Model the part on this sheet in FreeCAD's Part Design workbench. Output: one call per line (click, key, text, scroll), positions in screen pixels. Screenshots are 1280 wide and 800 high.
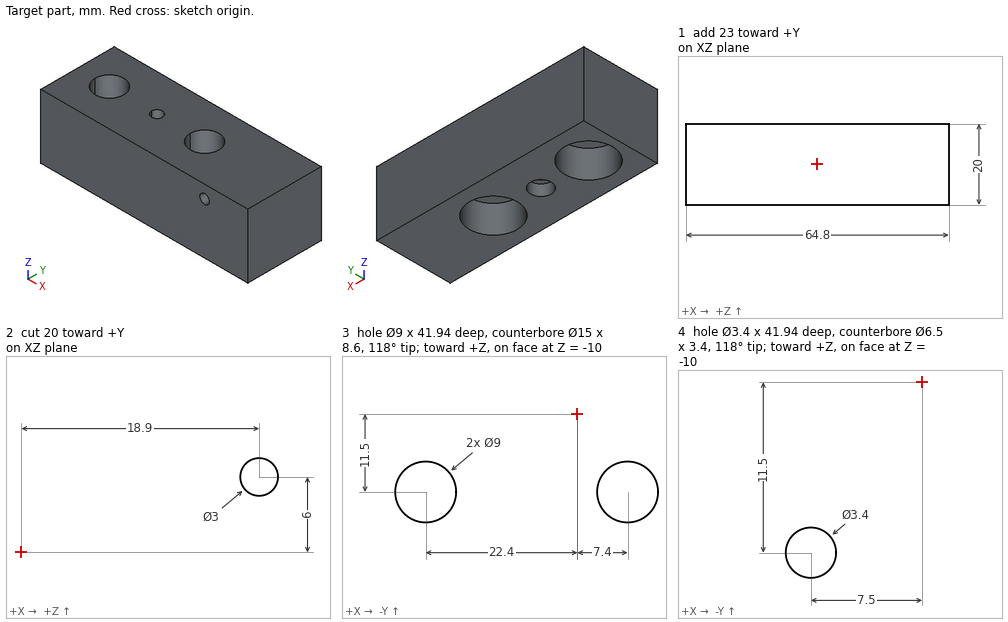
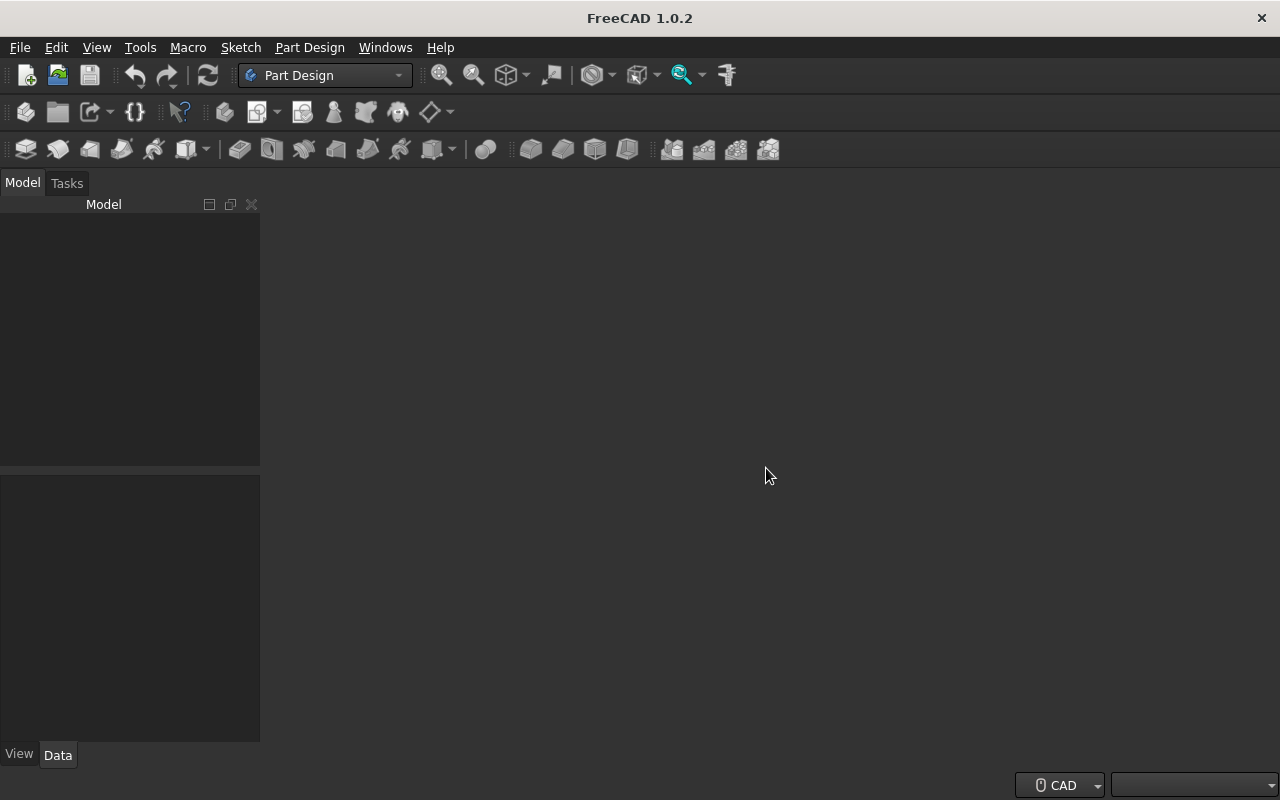
click(26, 76)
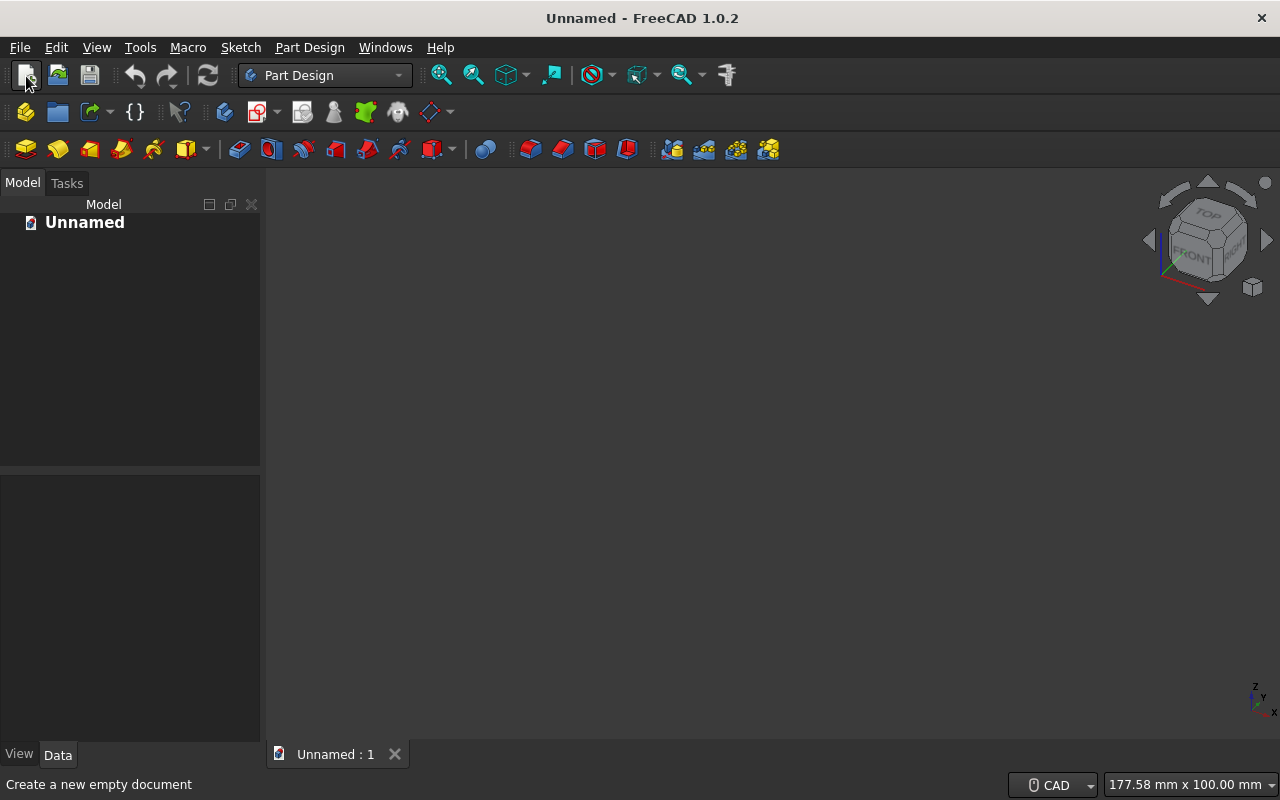
click(258, 112)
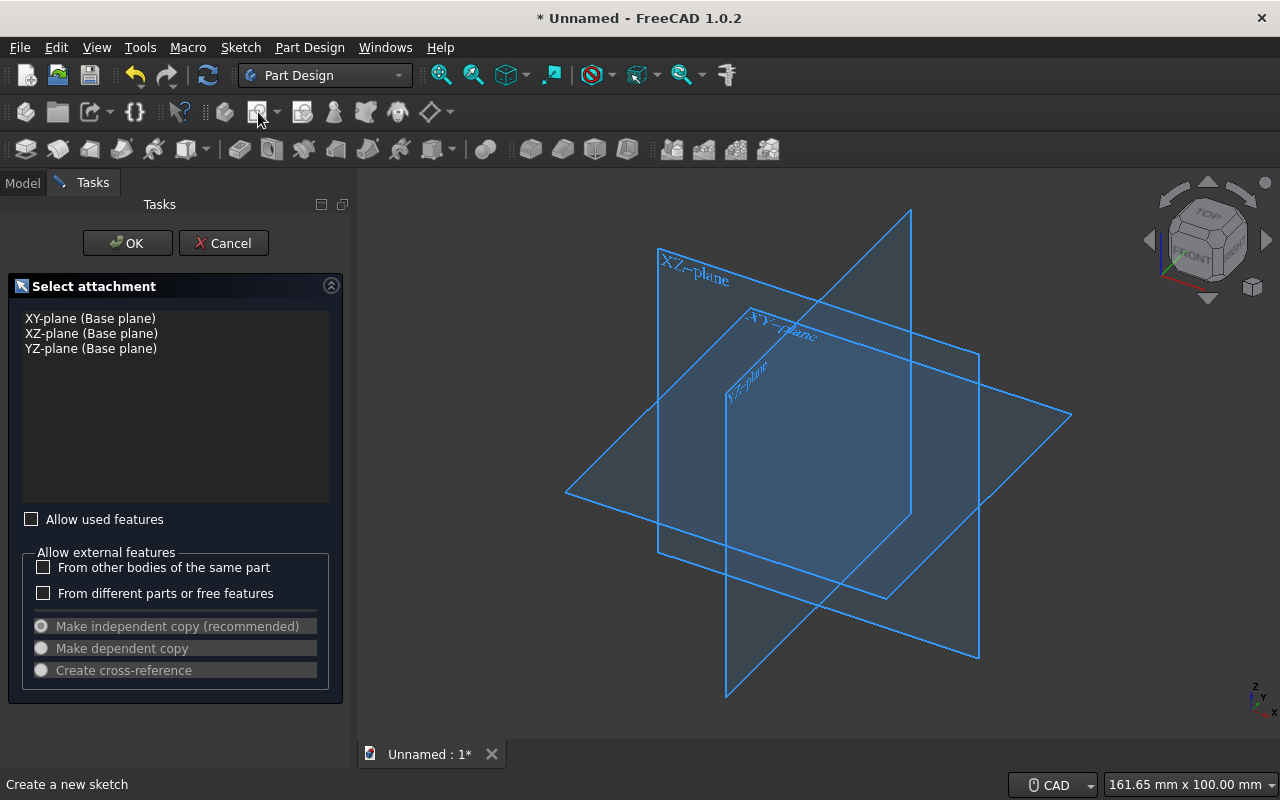
click(82, 334)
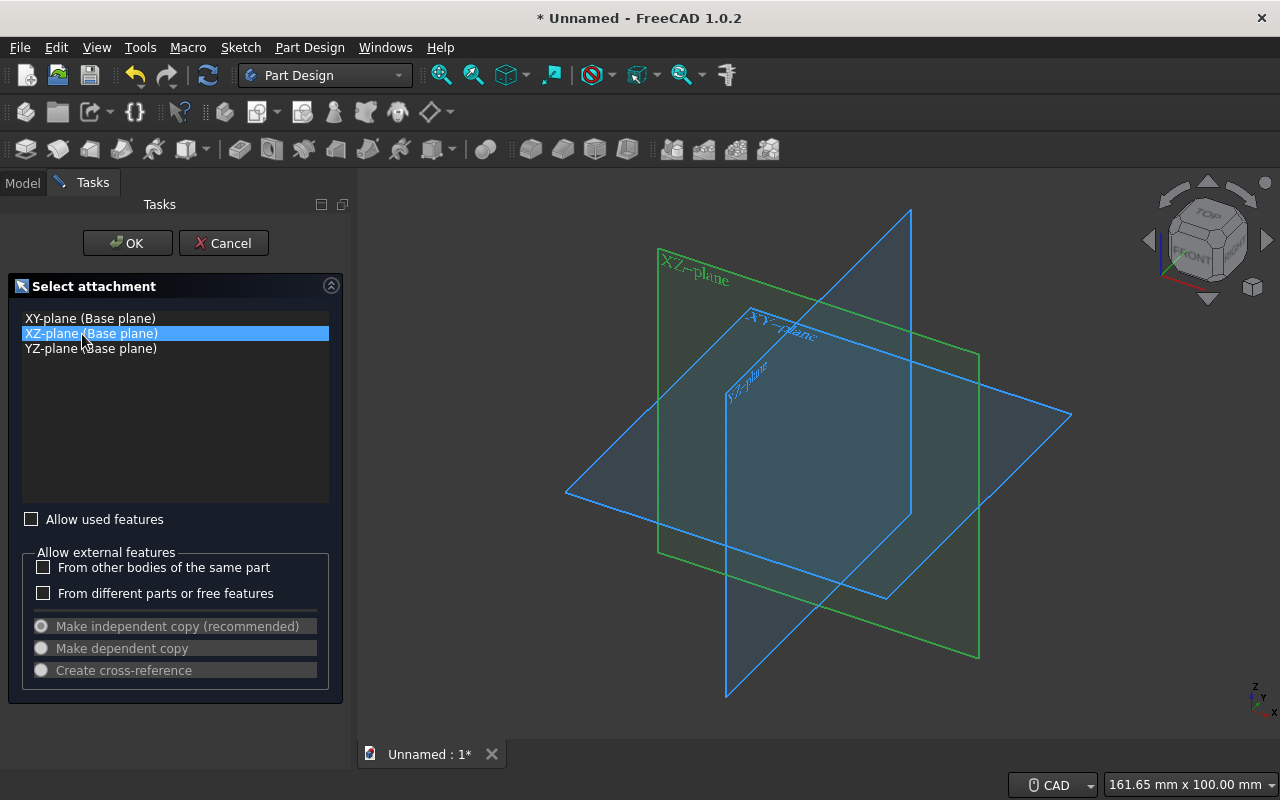
click(128, 243)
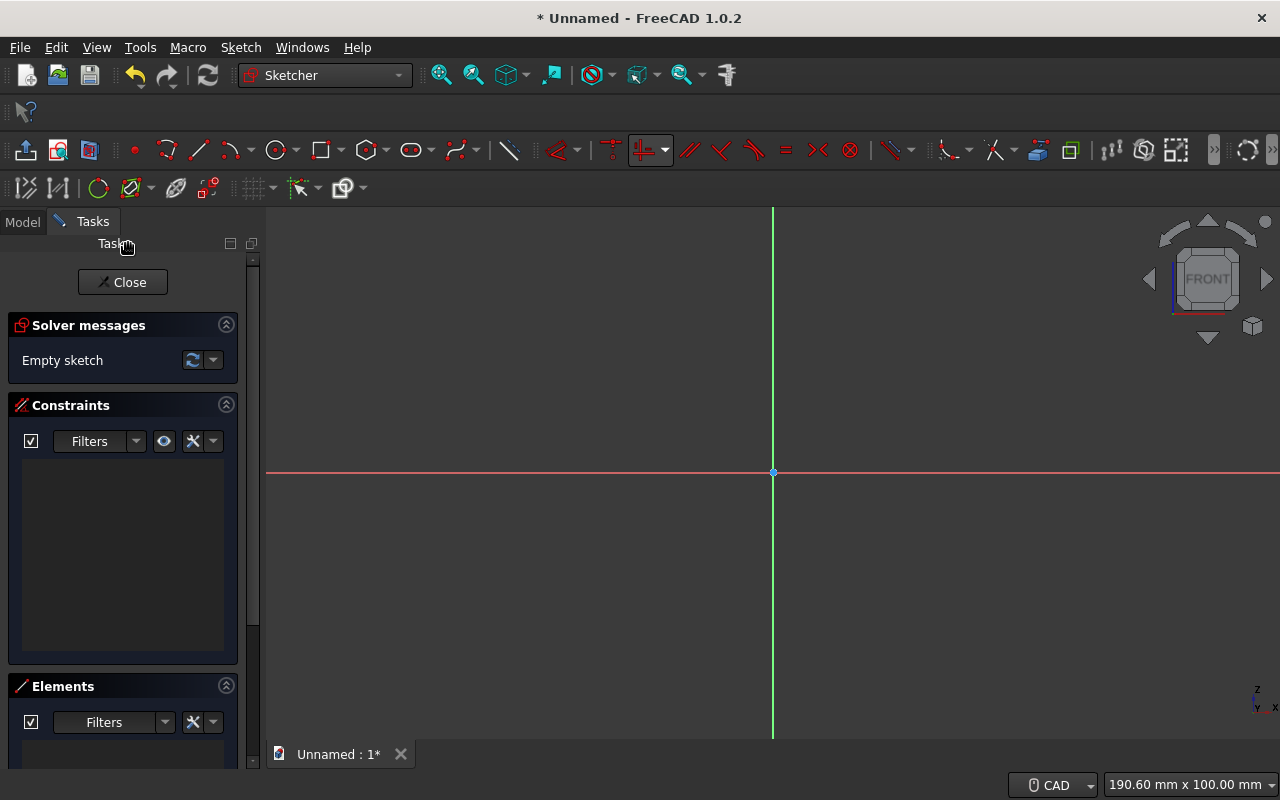
scroll(856, 473, up, 3)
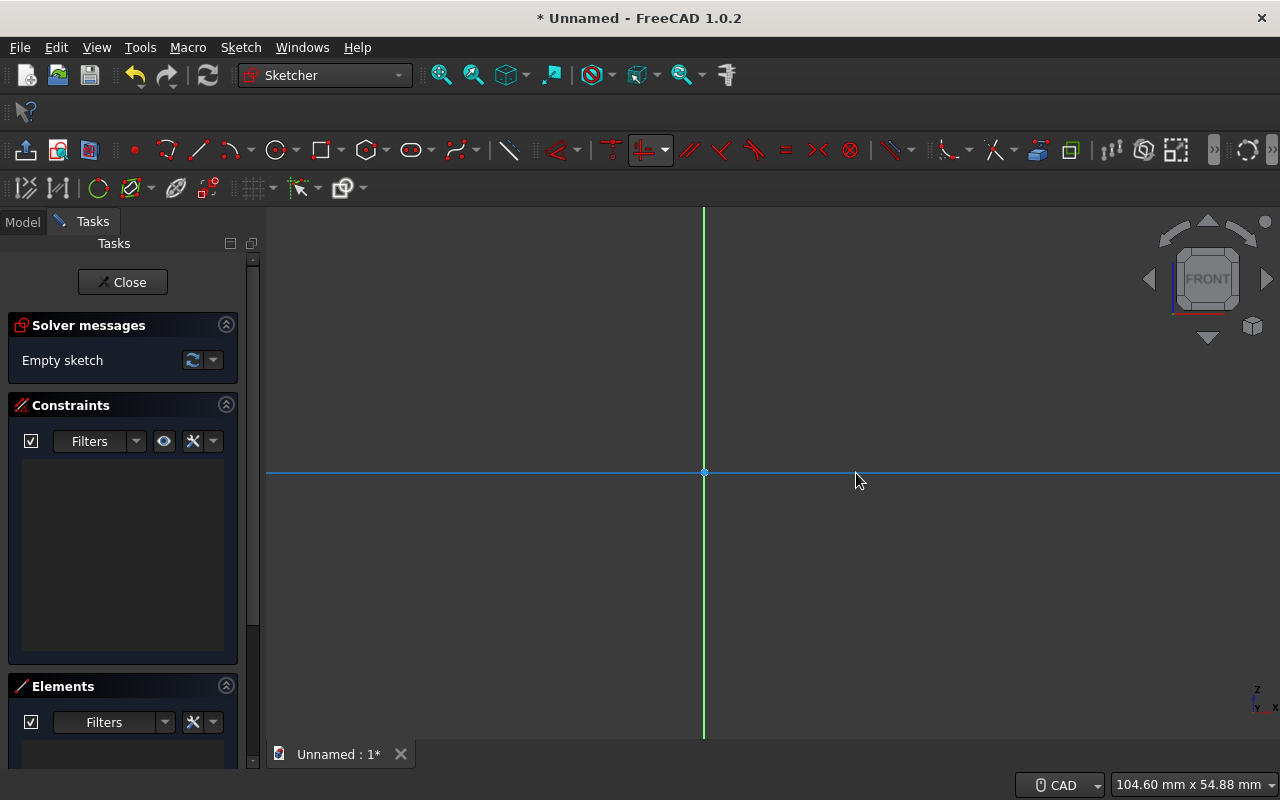
key(g)
key(v)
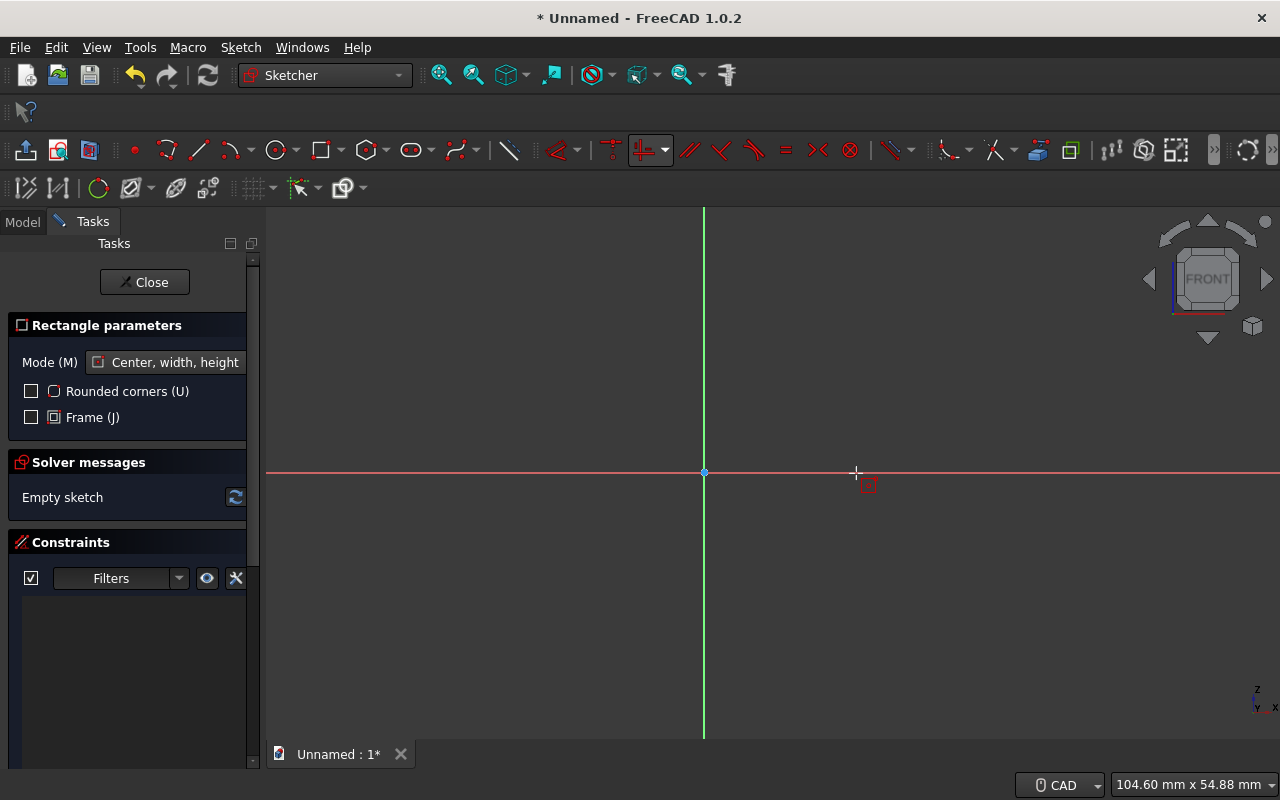
click(704, 473)
move(1018, 376)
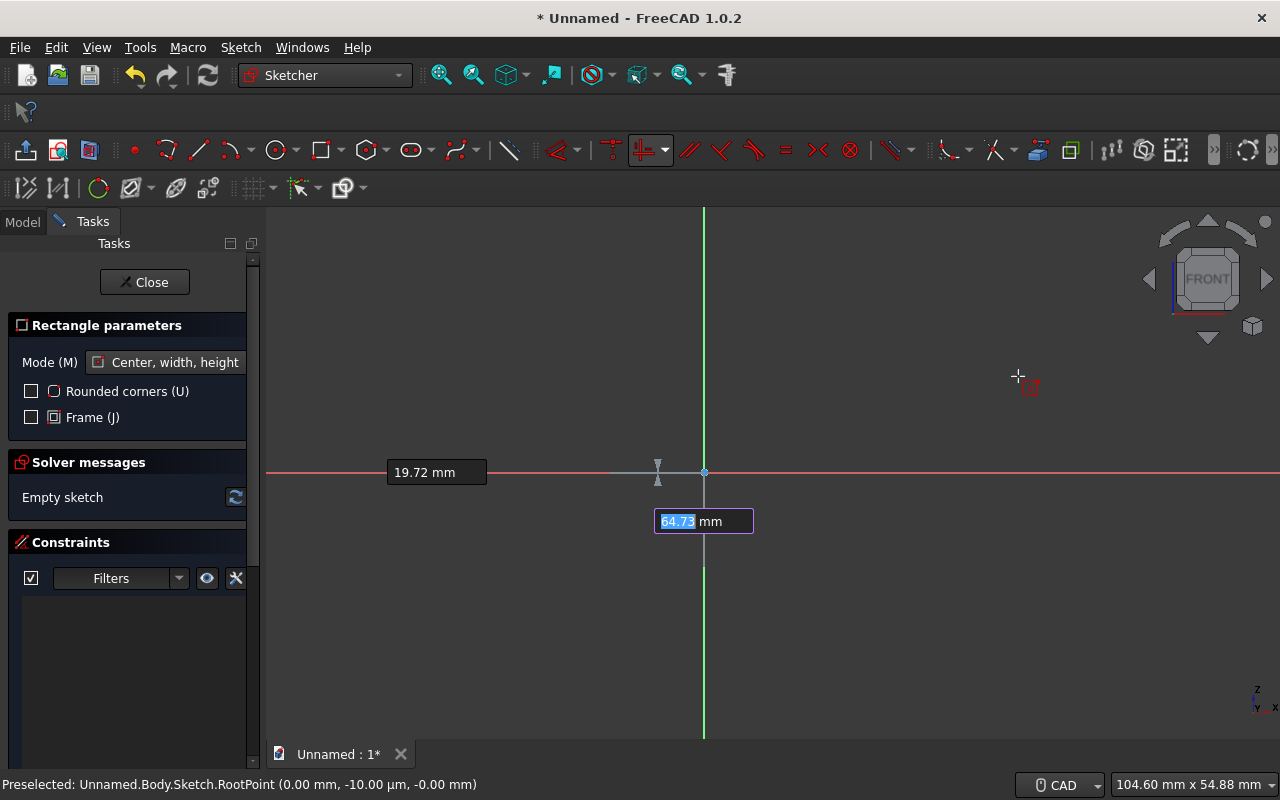
text(64.8)
key(Tab)
text(20)
key(Return)
key(Escape)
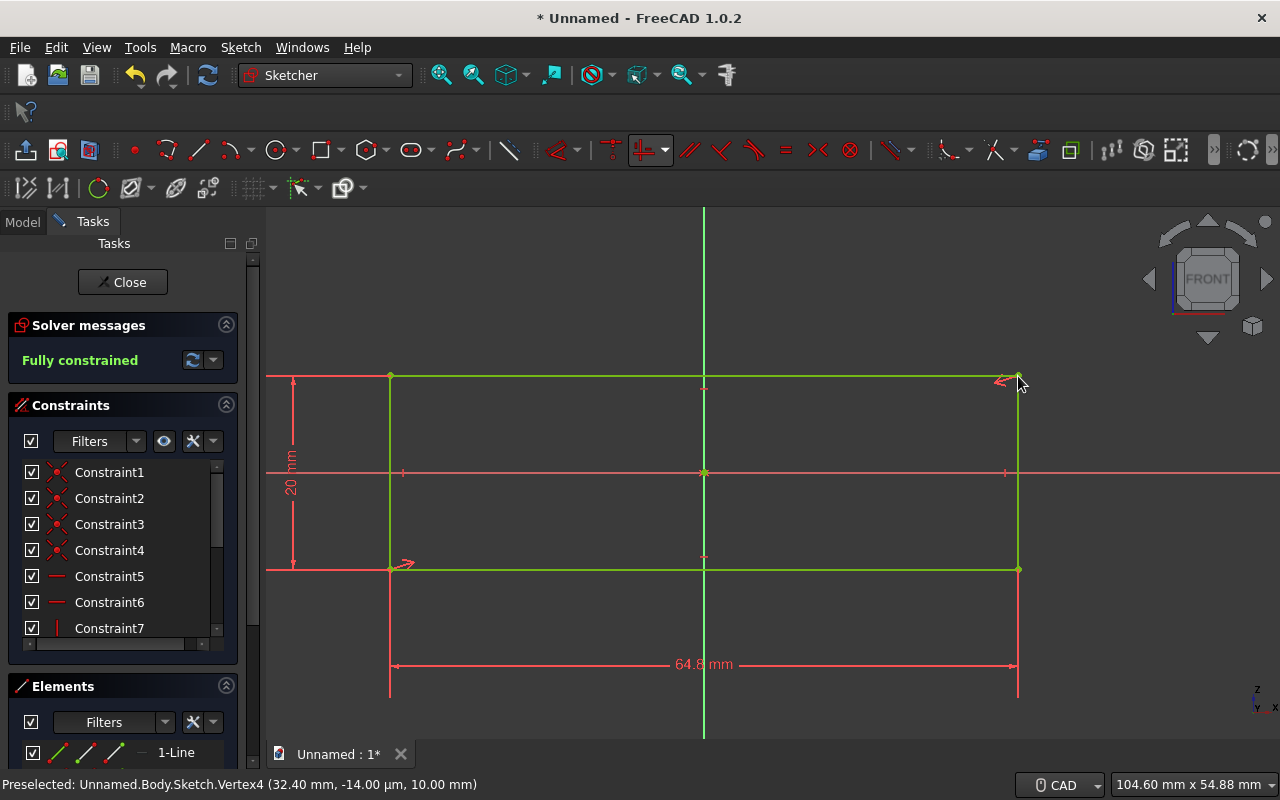
click(123, 282)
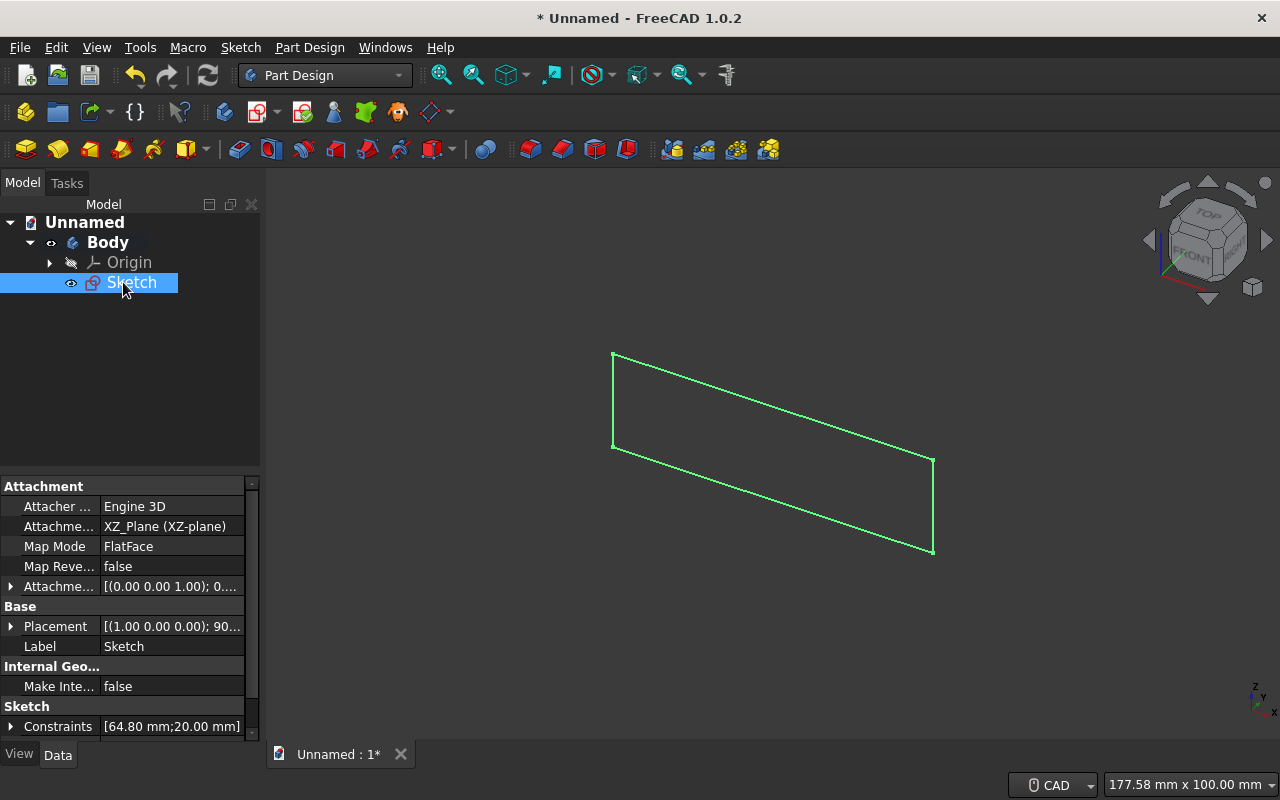
click(26, 150)